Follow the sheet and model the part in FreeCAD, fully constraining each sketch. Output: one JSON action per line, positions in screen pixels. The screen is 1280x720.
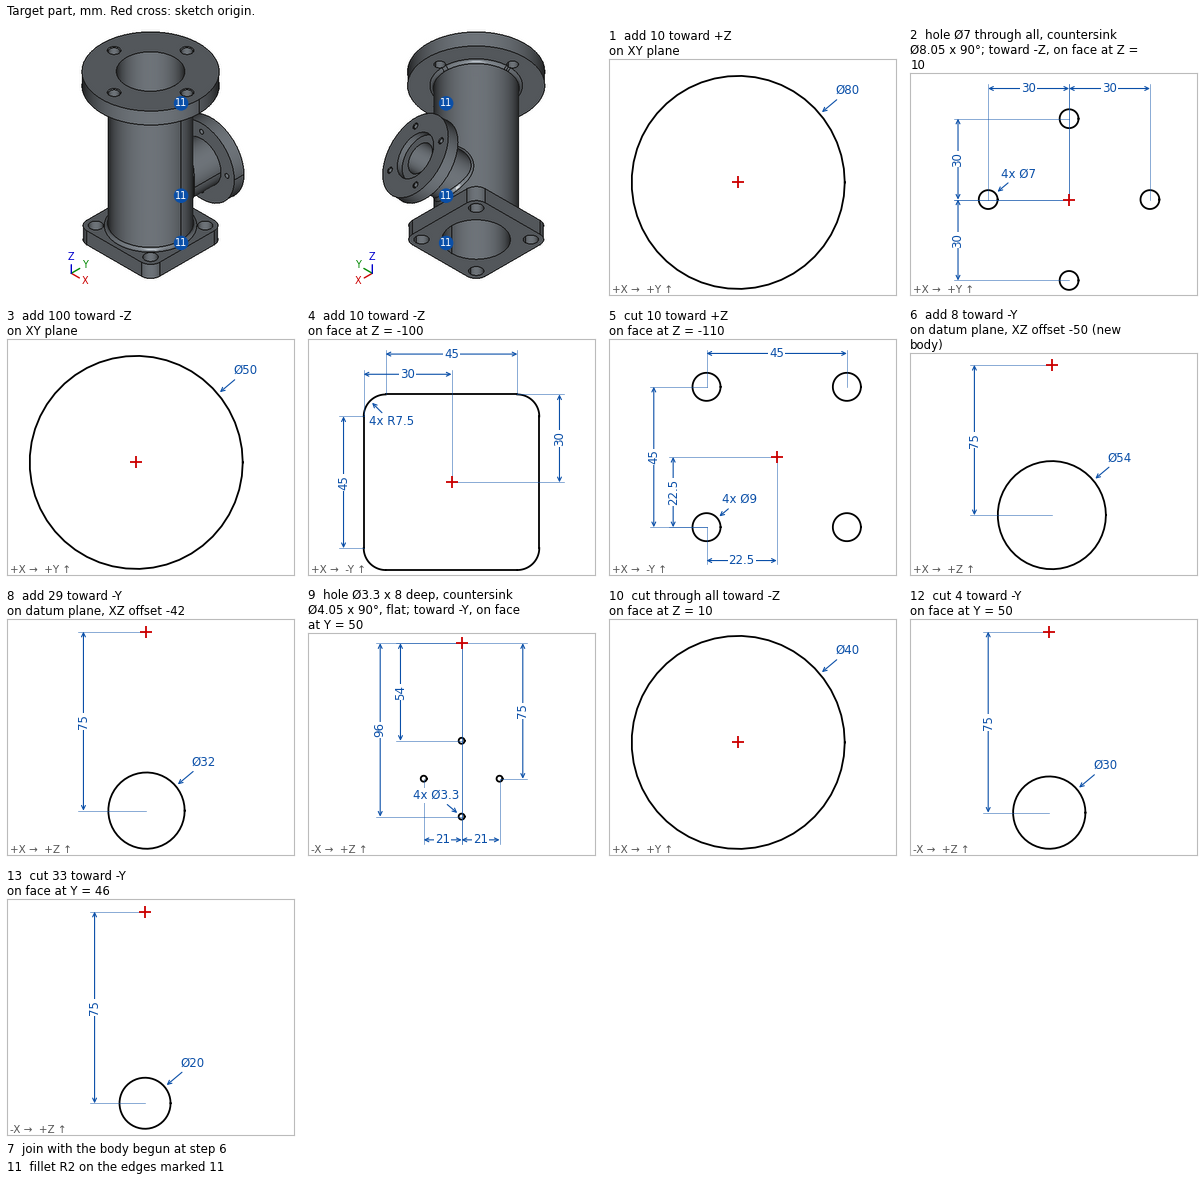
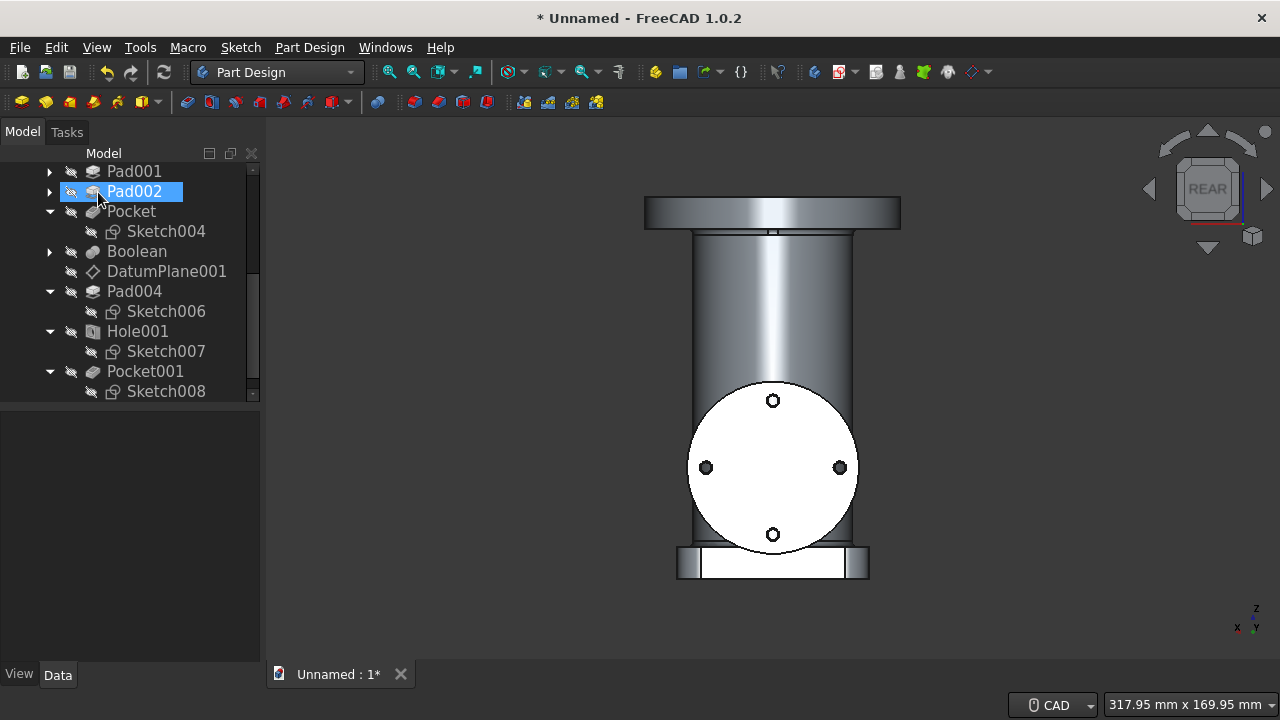
{"action": "left_click", "coordinate": [773, 467]}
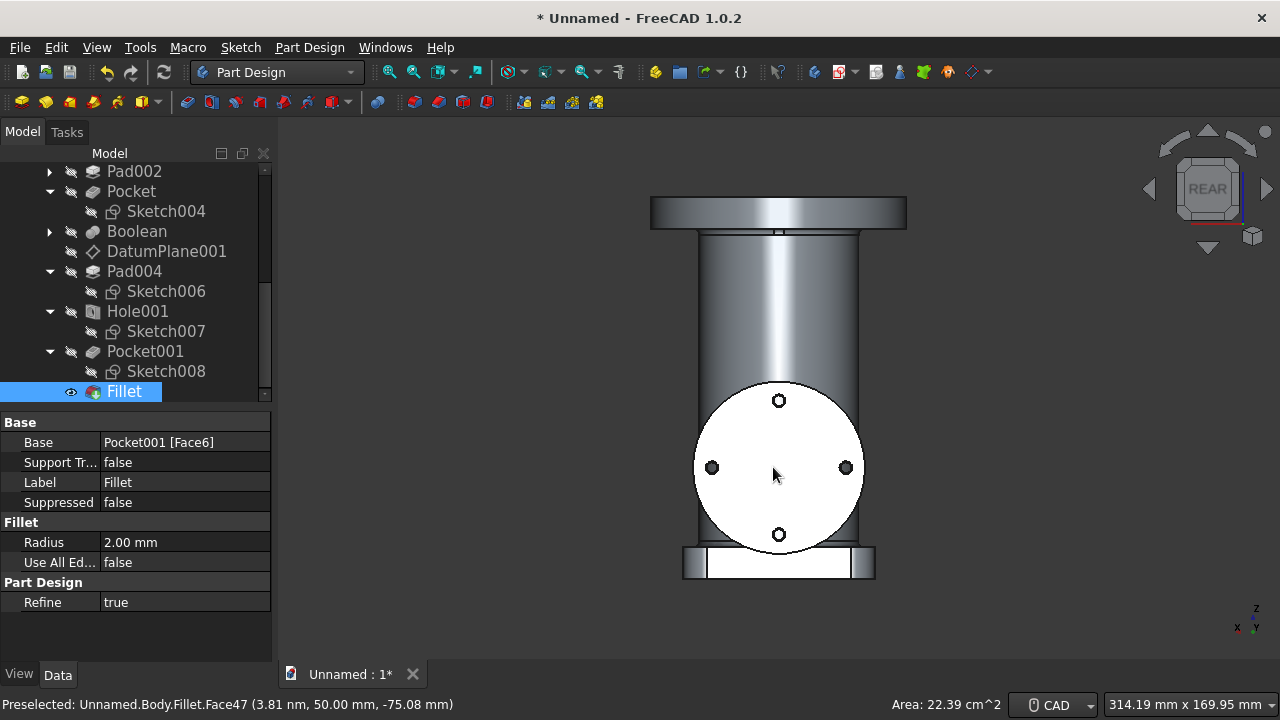
{"action": "left_click", "coordinate": [840, 72]}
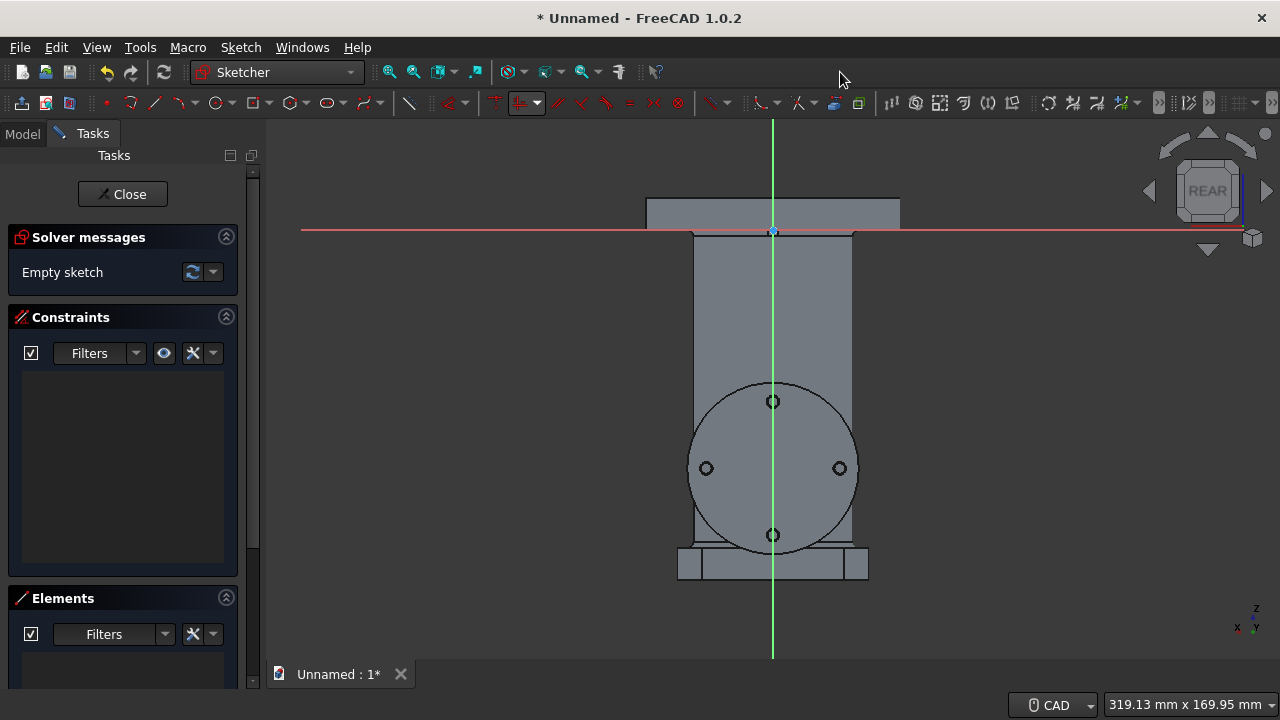
{"action": "scroll", "coordinate": [803, 503], "scroll_direction": "up", "scroll_amount": 6}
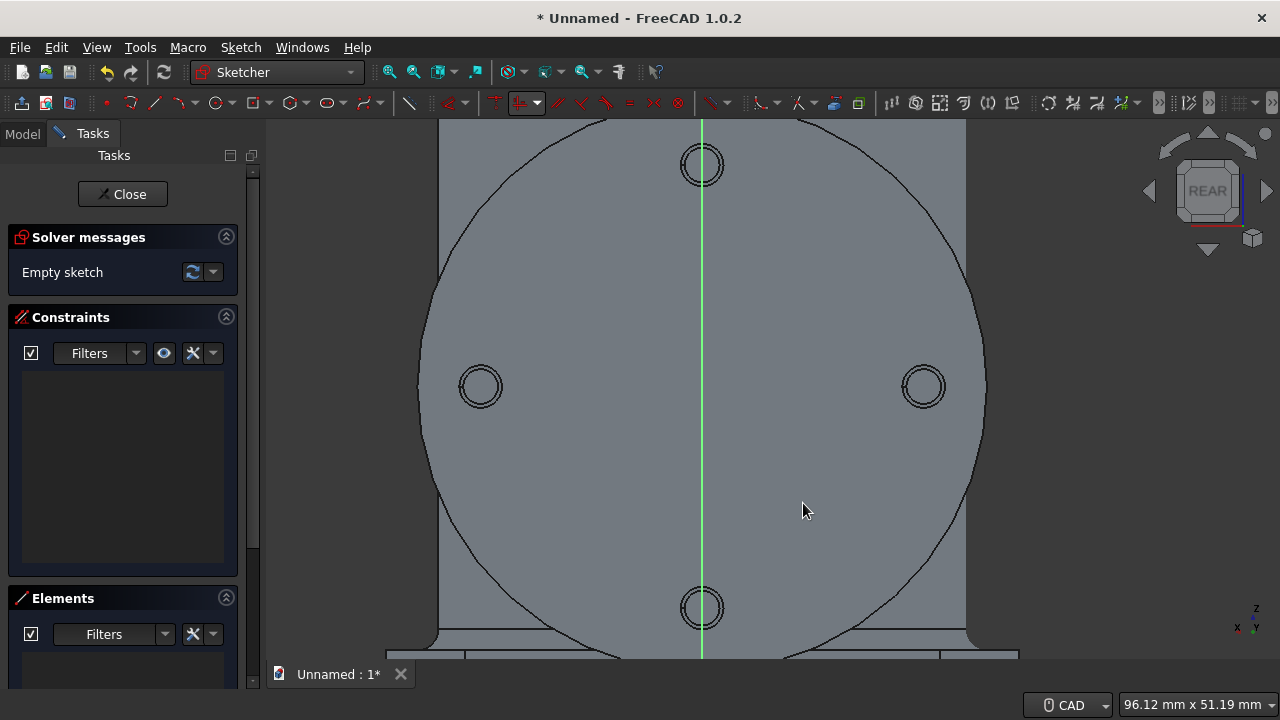
{"action": "left_click", "coordinate": [216, 104]}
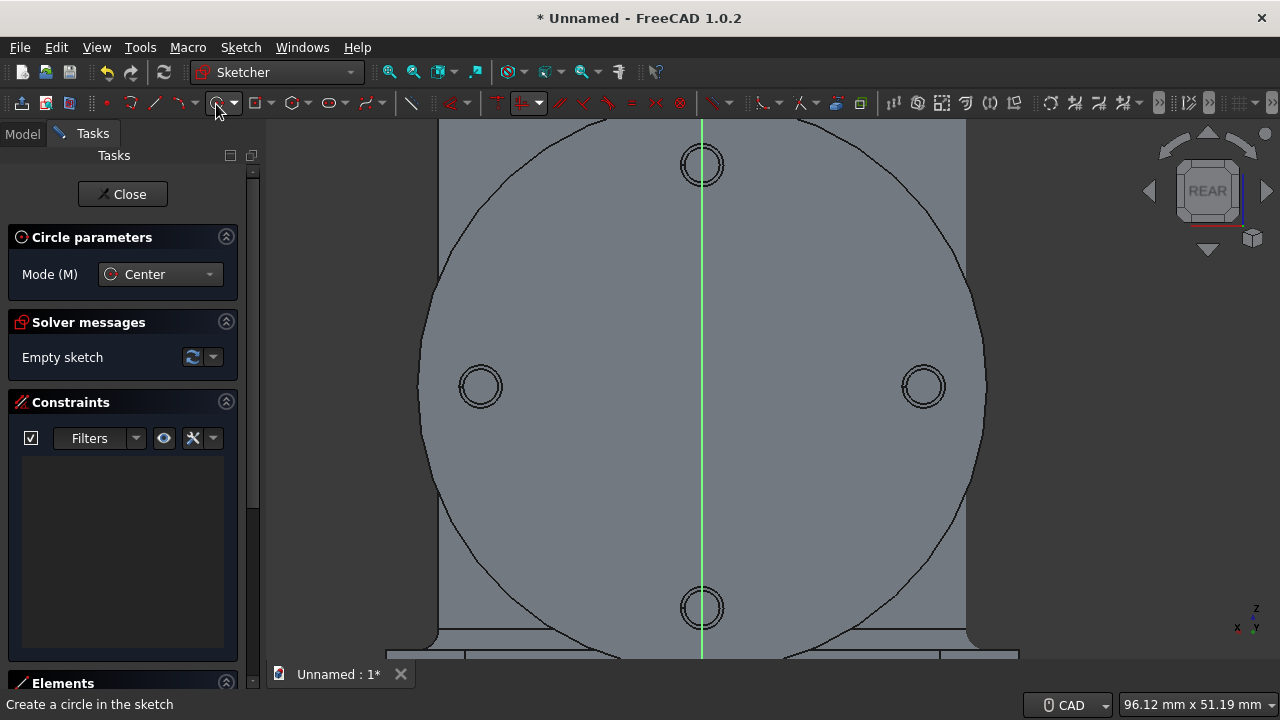
{"action": "left_click", "coordinate": [702, 387]}
{"action": "mouse_move", "coordinate": [814, 275]}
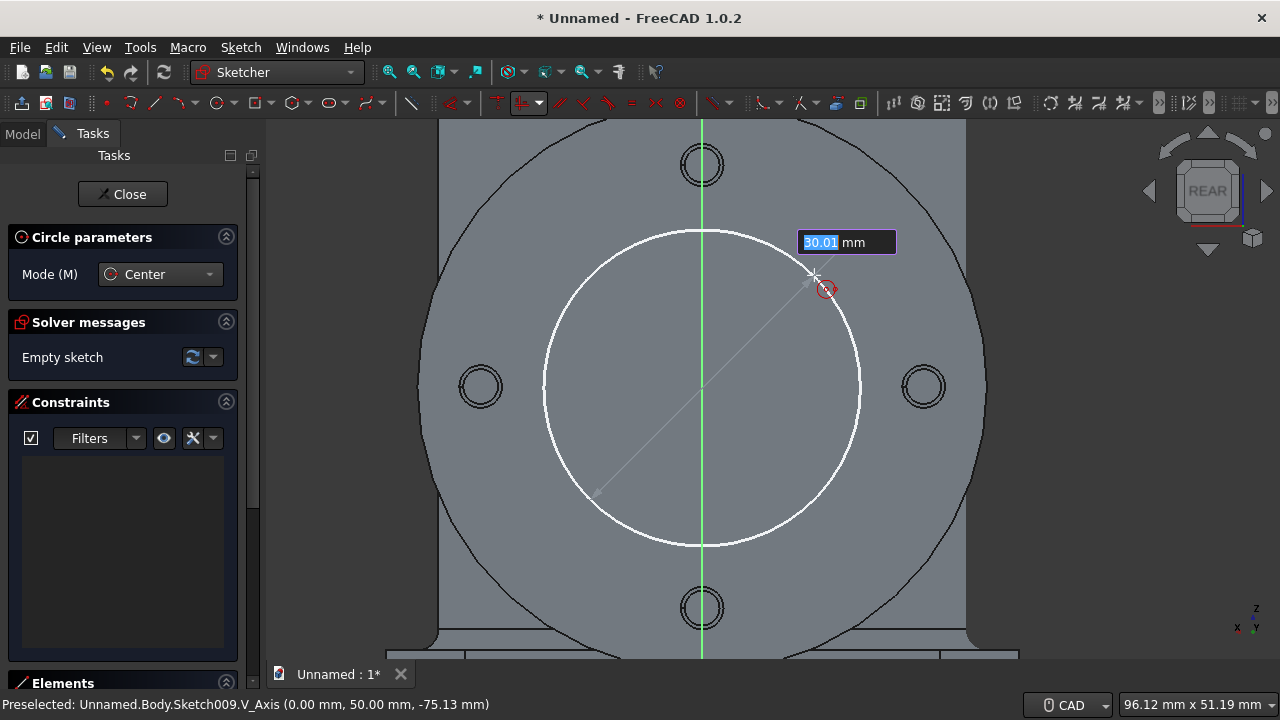
{"action": "type", "text": "30"}
{"action": "key", "text": "Return"}
{"action": "key", "text": "Escape"}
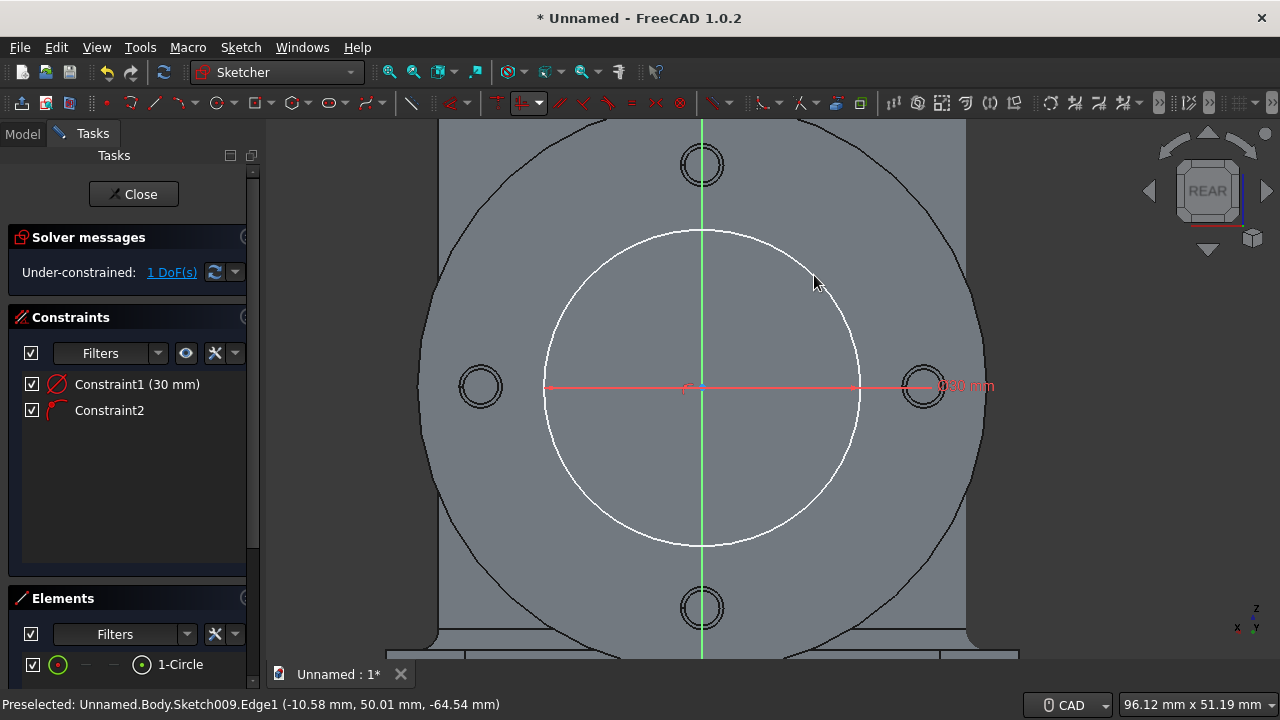
{"action": "left_click", "coordinate": [450, 104]}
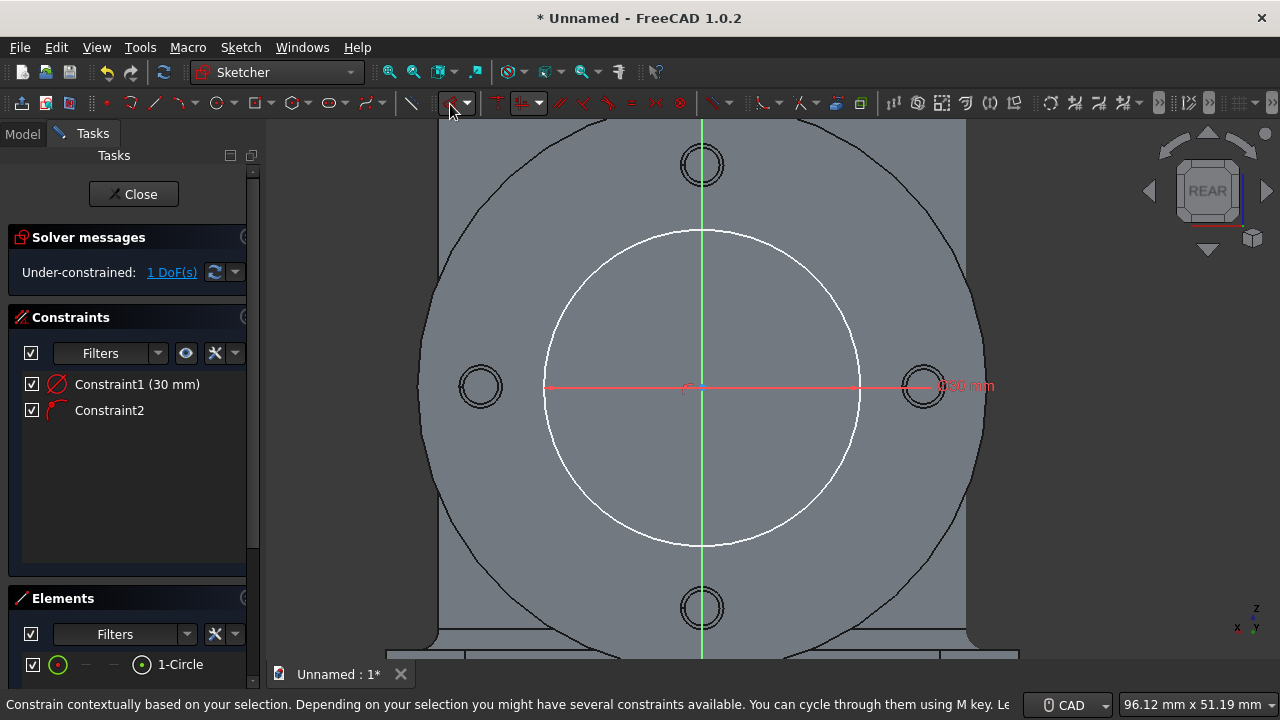
{"action": "left_click", "coordinate": [702, 388]}
{"action": "left_click", "coordinate": [736, 267]}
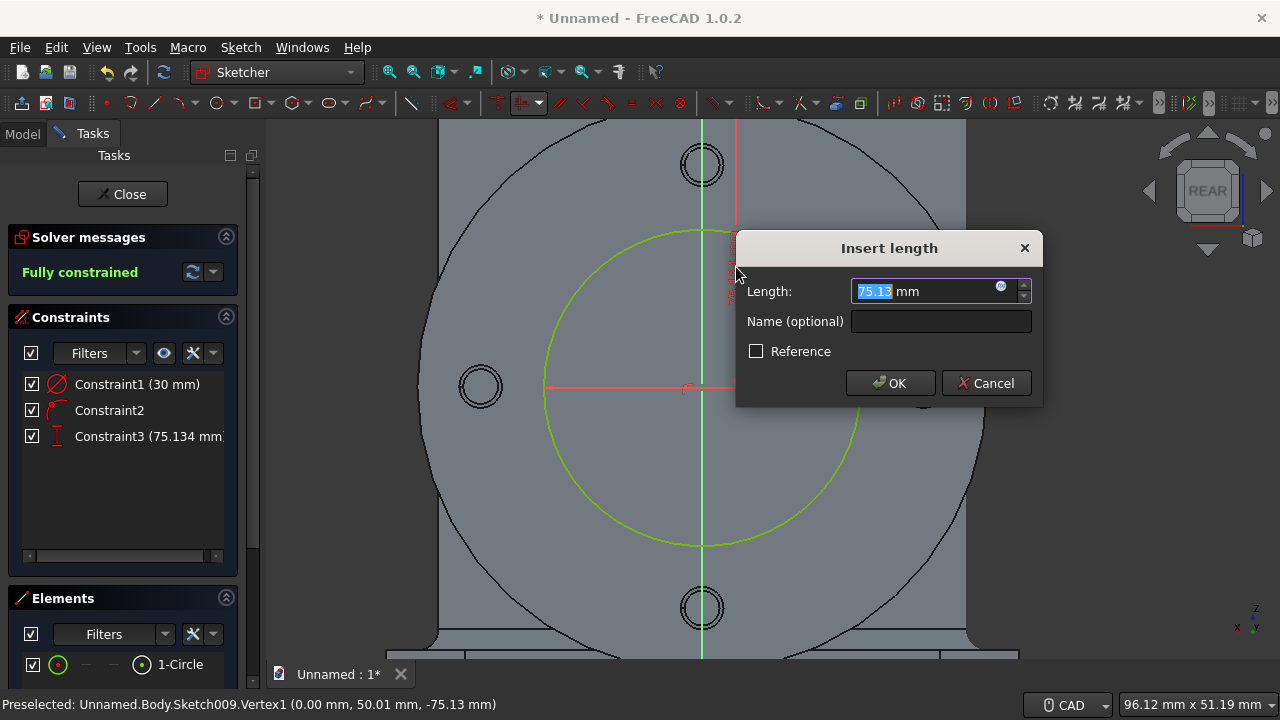
{"action": "type", "text": "75"}
{"action": "key", "text": "Return"}
{"action": "key", "text": "Escape"}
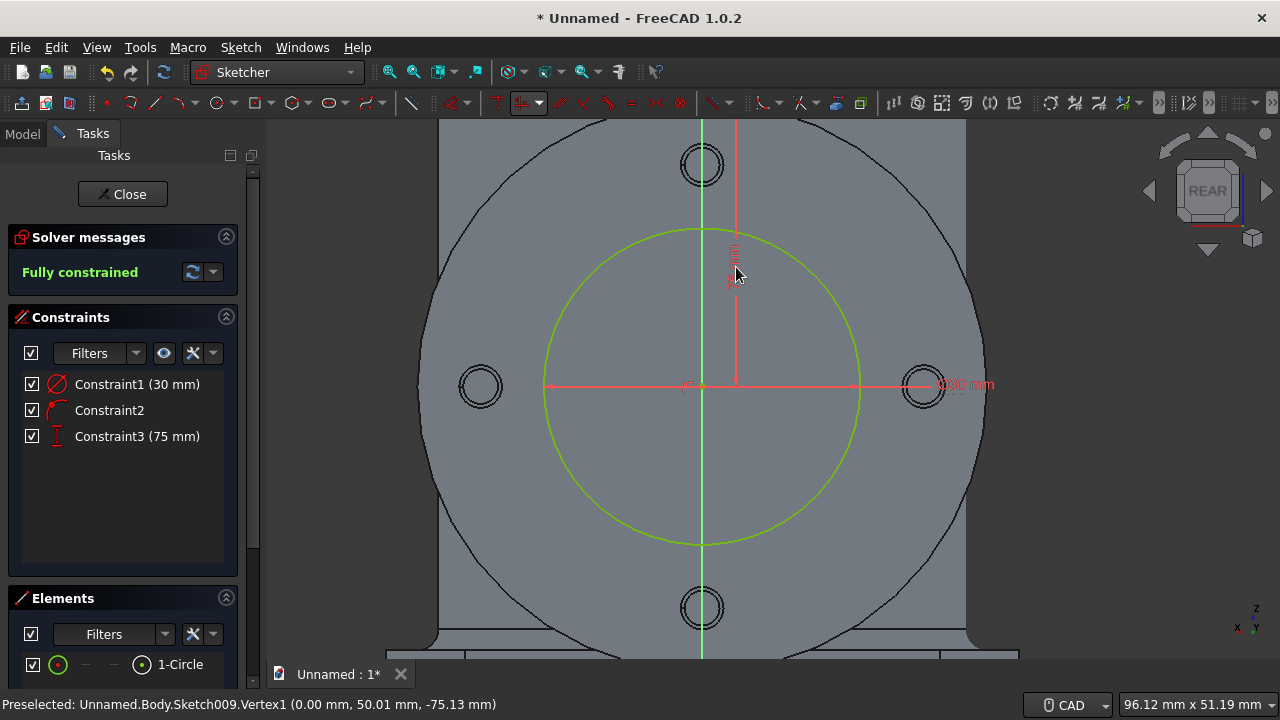
{"action": "left_click", "coordinate": [123, 194]}